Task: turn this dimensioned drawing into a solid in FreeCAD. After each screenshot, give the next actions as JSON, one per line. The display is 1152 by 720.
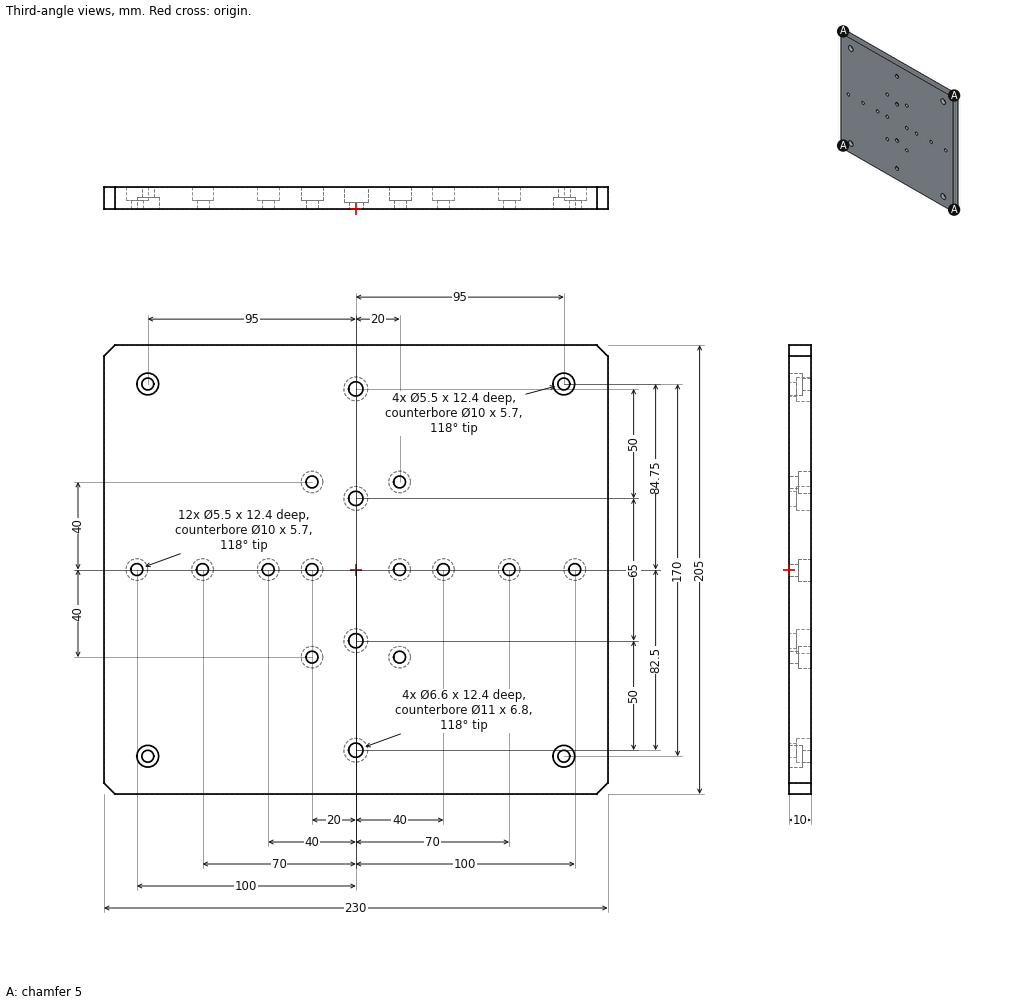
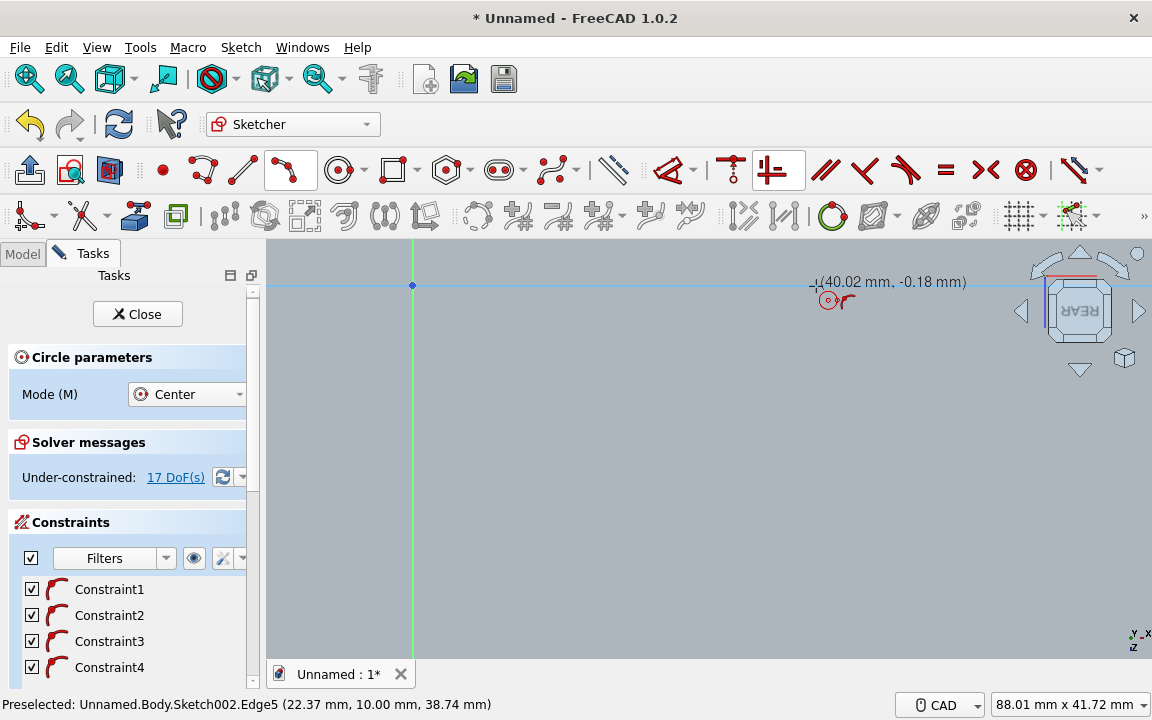
{"action": "scroll", "coordinate": [715, 502], "scroll_direction": "down", "scroll_amount": 7}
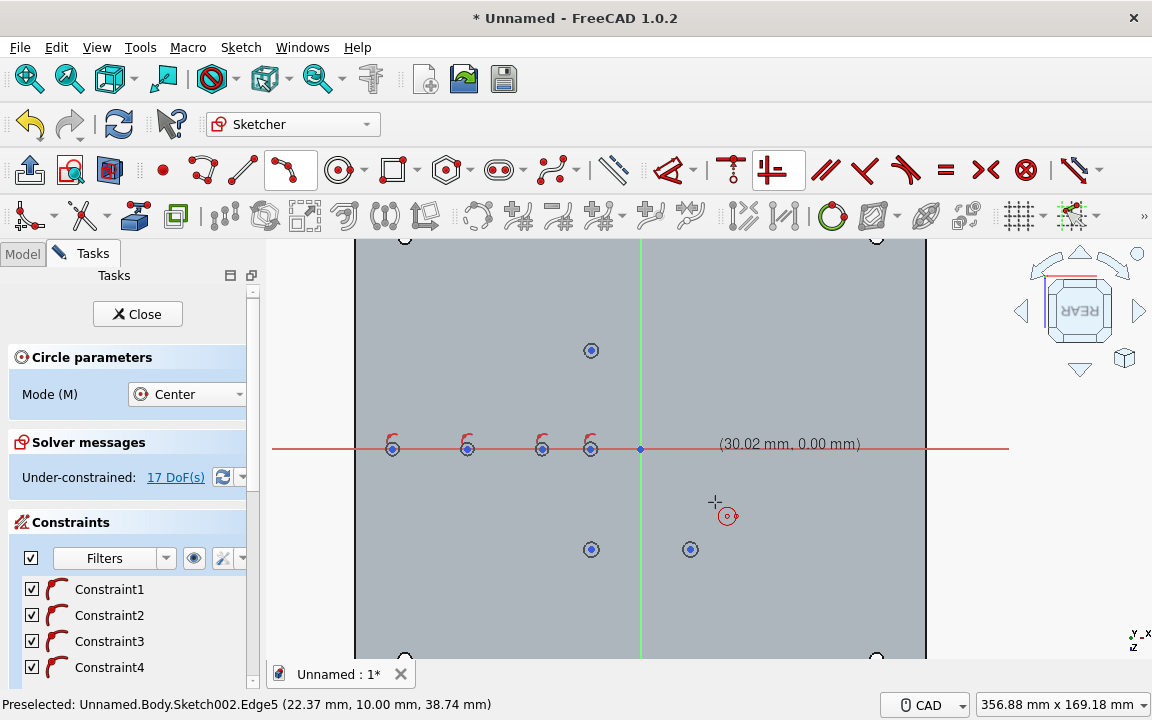
{"action": "left_click", "coordinate": [740, 449]}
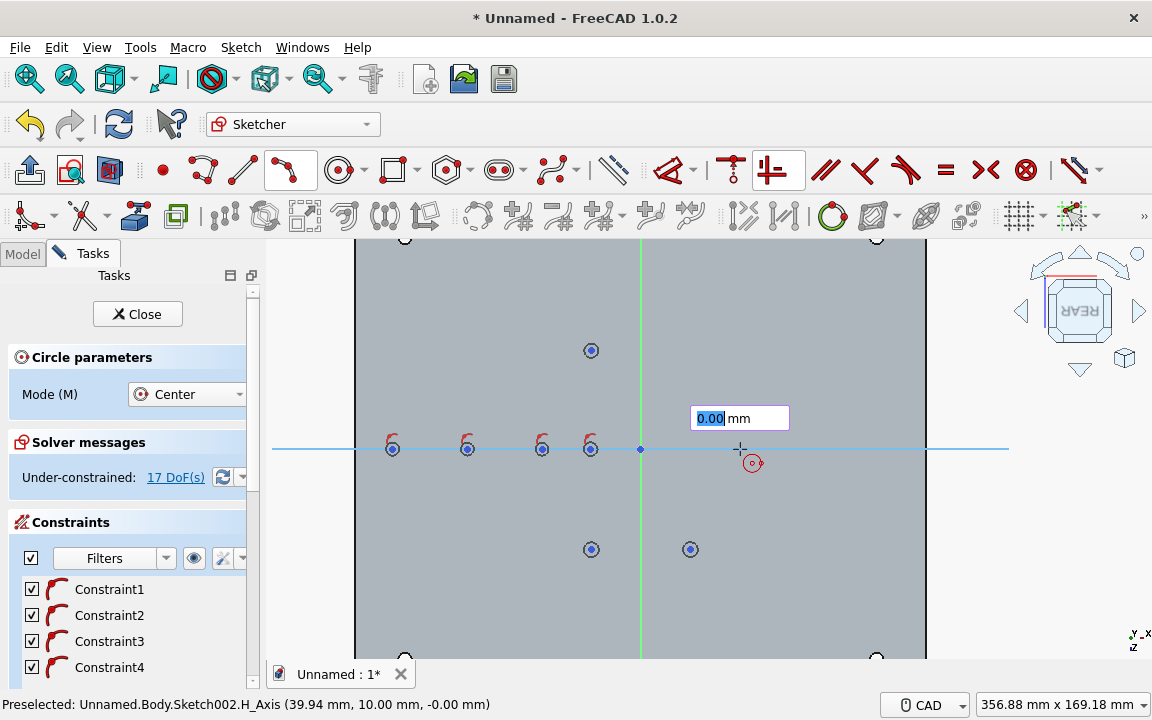
{"action": "scroll", "coordinate": [742, 443], "scroll_direction": "up", "scroll_amount": 5}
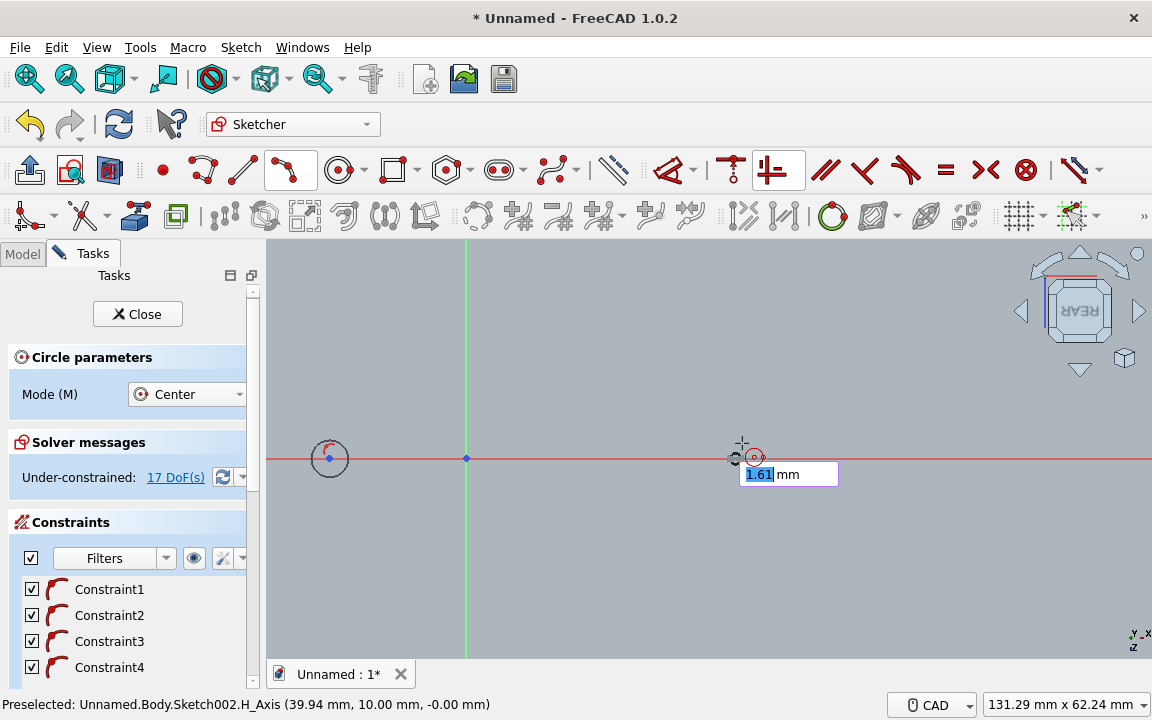
{"action": "left_click", "coordinate": [742, 441]}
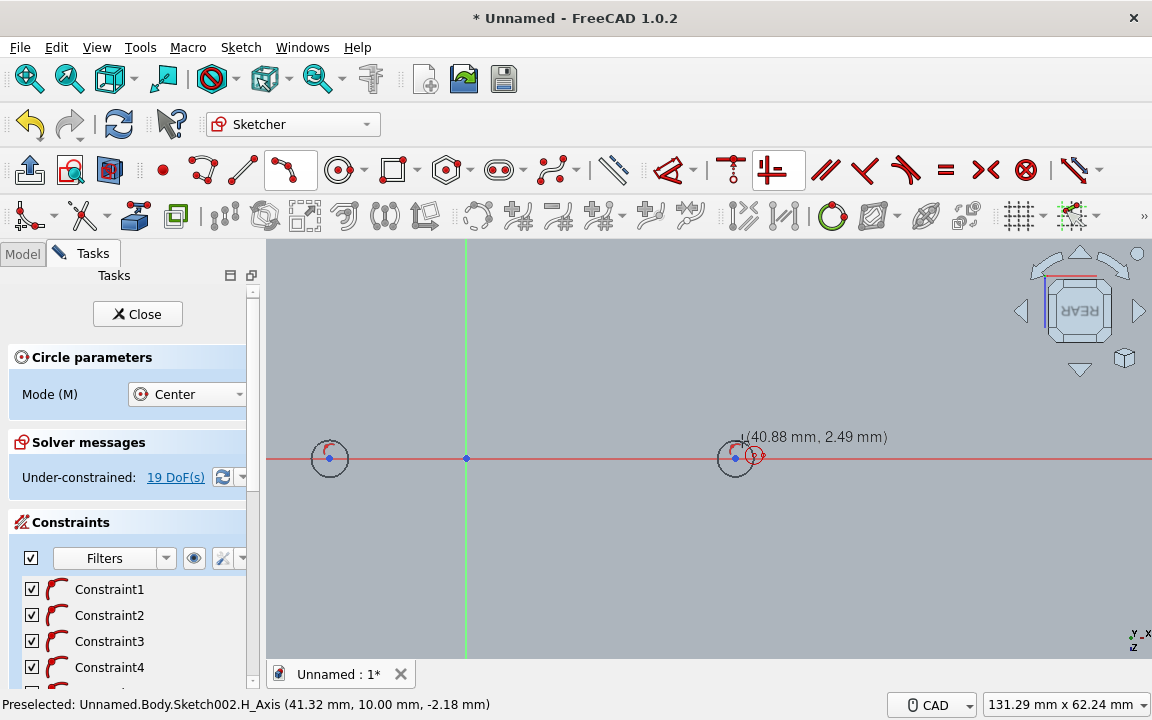
{"action": "scroll", "coordinate": [601, 459], "scroll_direction": "up", "scroll_amount": 2}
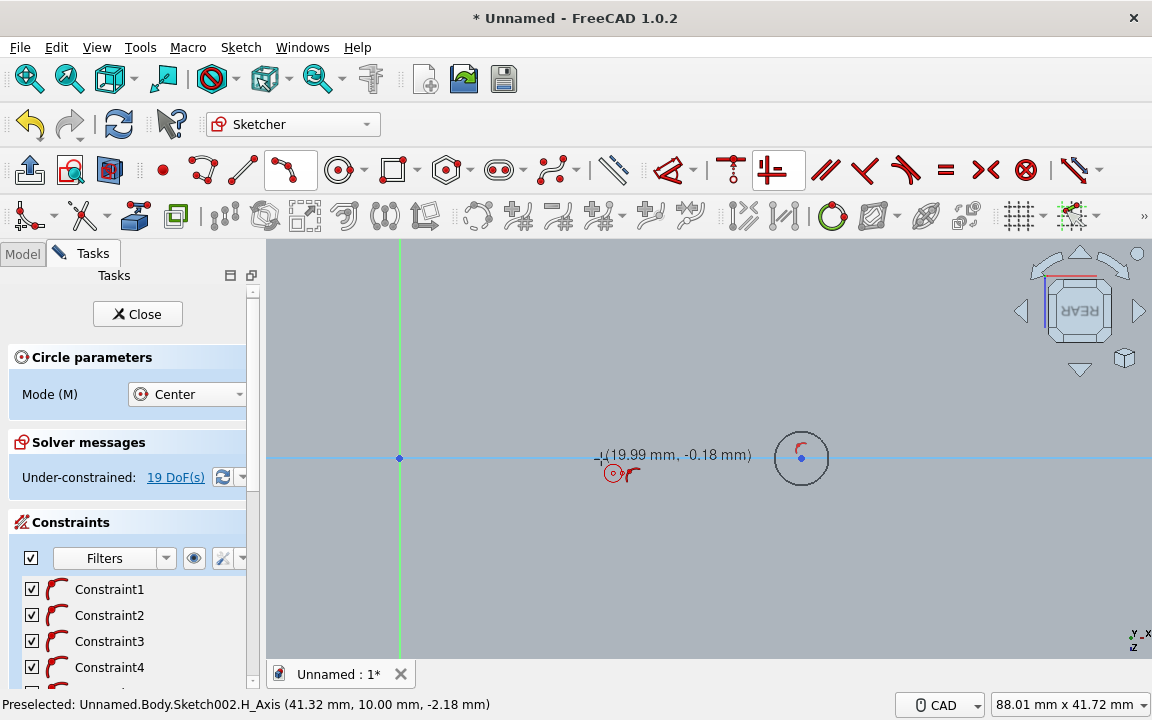
{"action": "scroll", "coordinate": [719, 446], "scroll_direction": "down", "scroll_amount": 7}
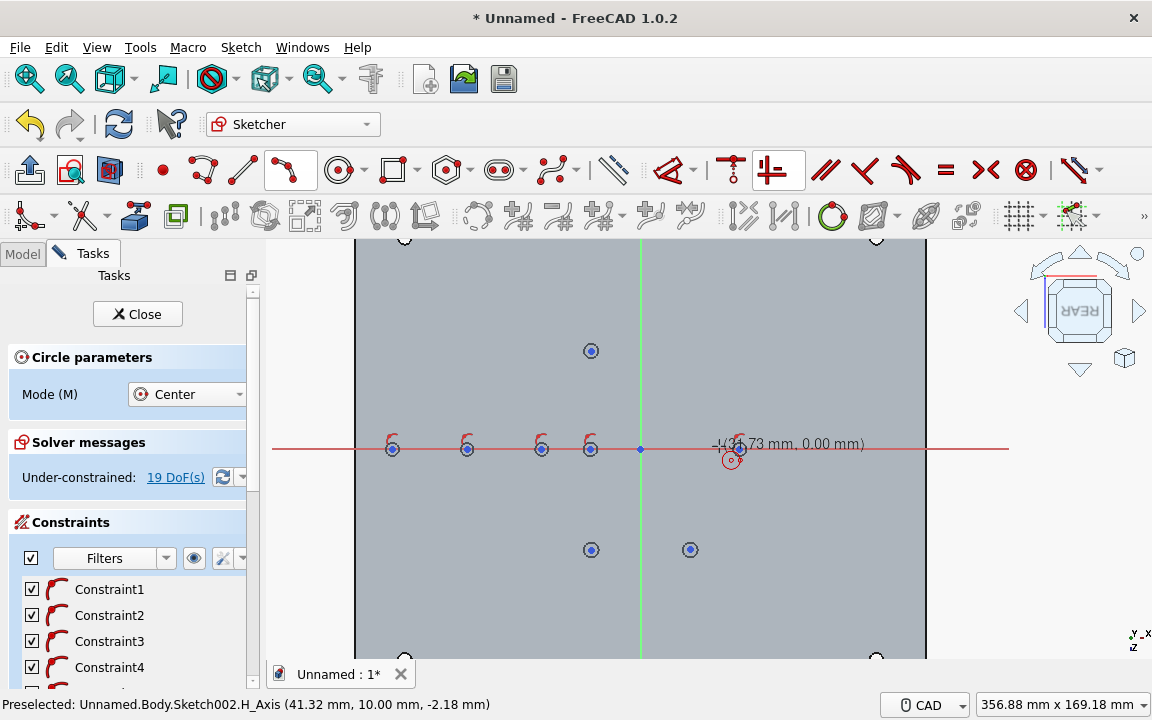
{"action": "left_click", "coordinate": [690, 449]}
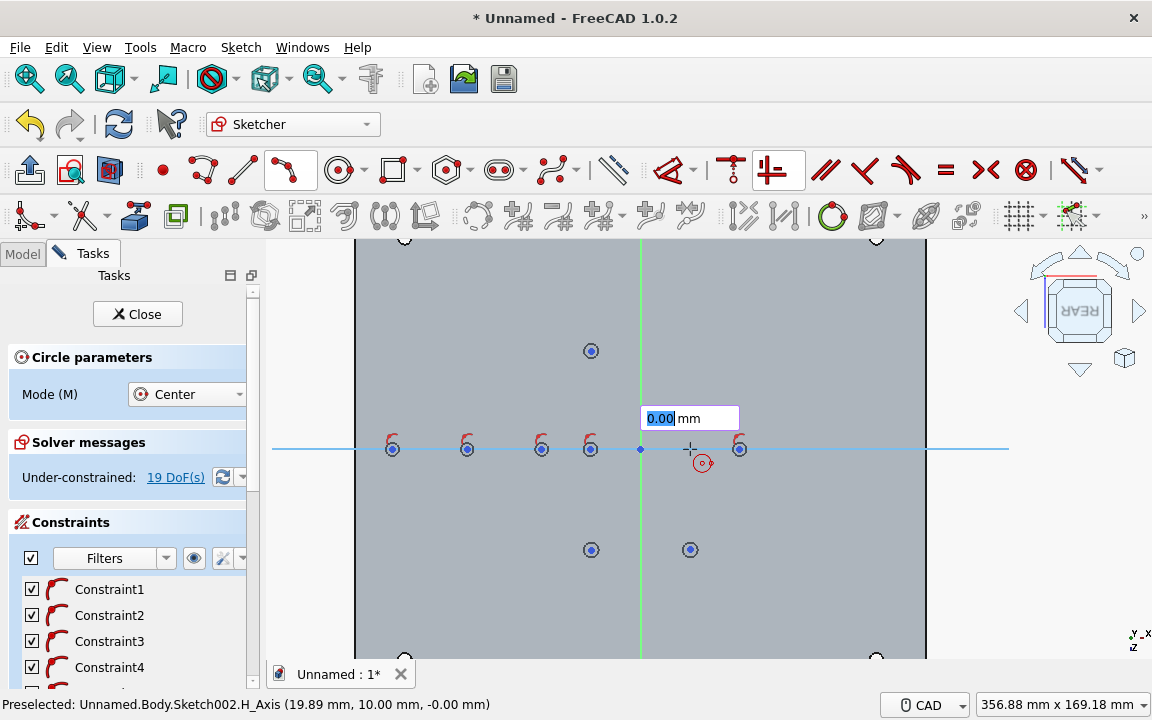
{"action": "scroll", "coordinate": [693, 443], "scroll_direction": "up", "scroll_amount": 5}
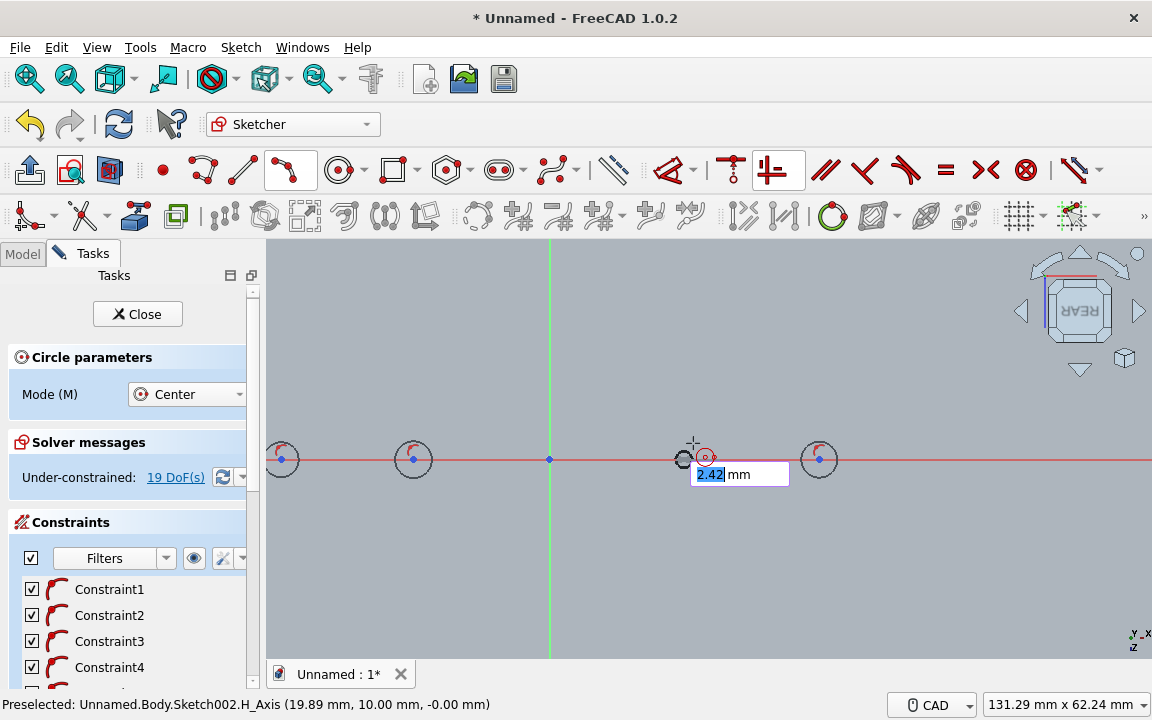
{"action": "left_click", "coordinate": [691, 442]}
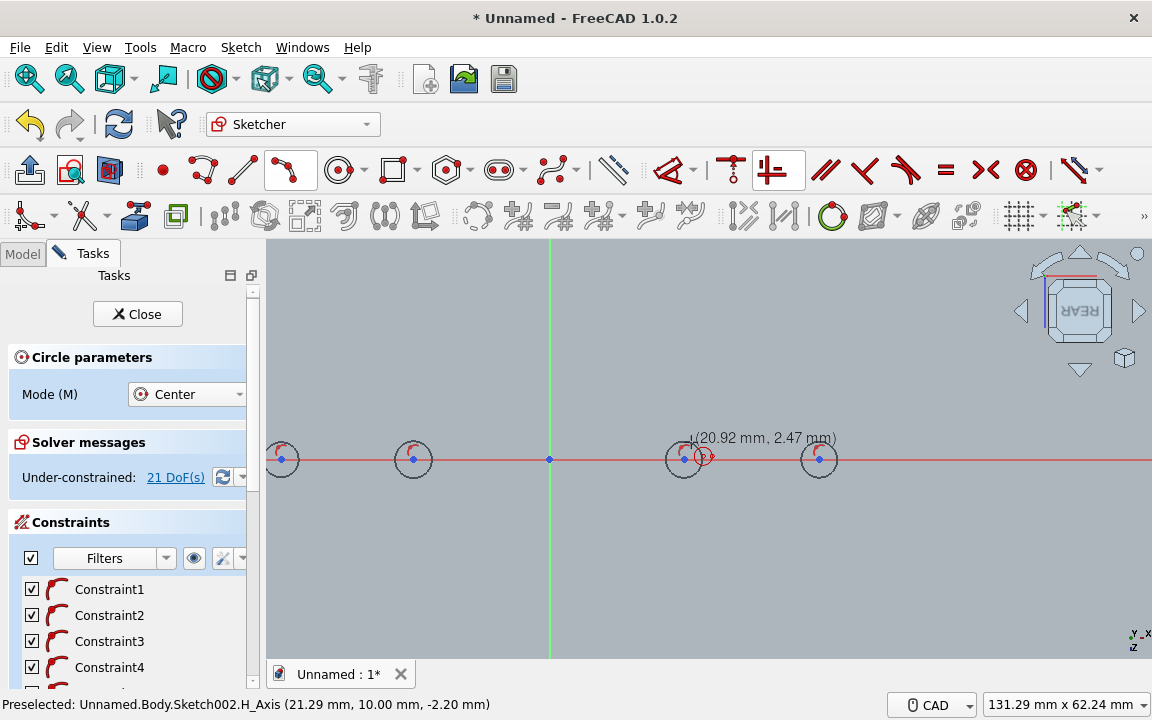
{"action": "scroll", "coordinate": [693, 443], "scroll_direction": "down", "scroll_amount": 5}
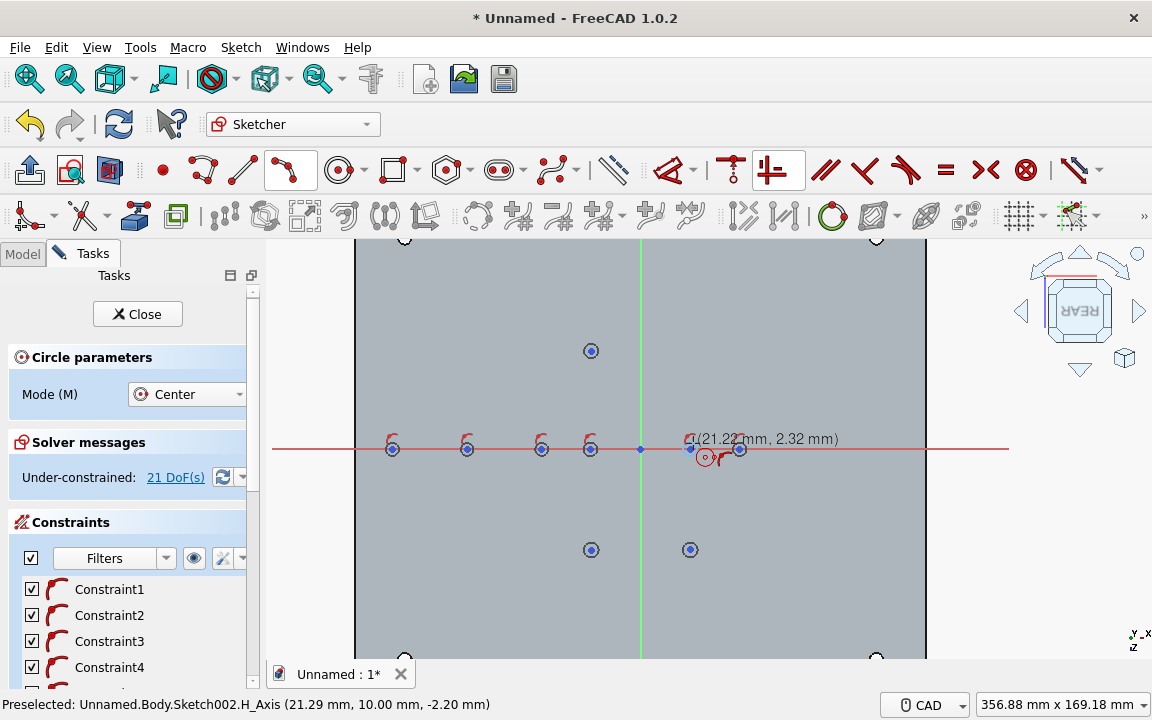
{"action": "scroll", "coordinate": [814, 449], "scroll_direction": "up", "scroll_amount": 7}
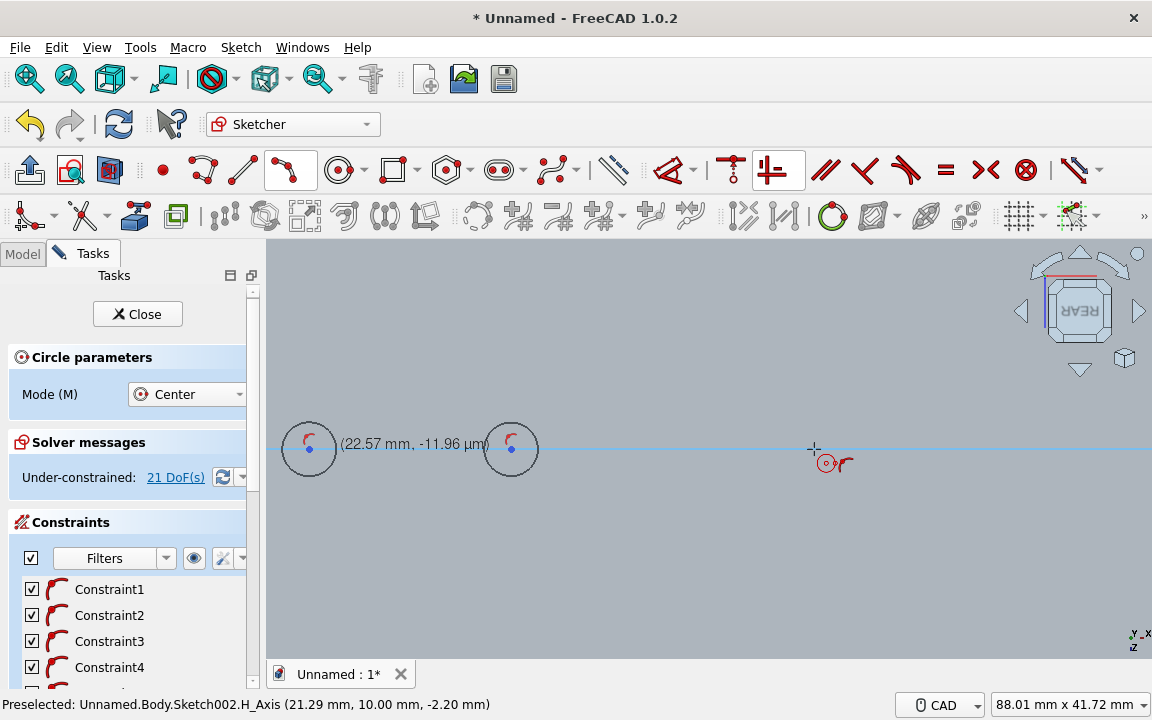
{"action": "scroll", "coordinate": [814, 449], "scroll_direction": "down", "scroll_amount": 7}